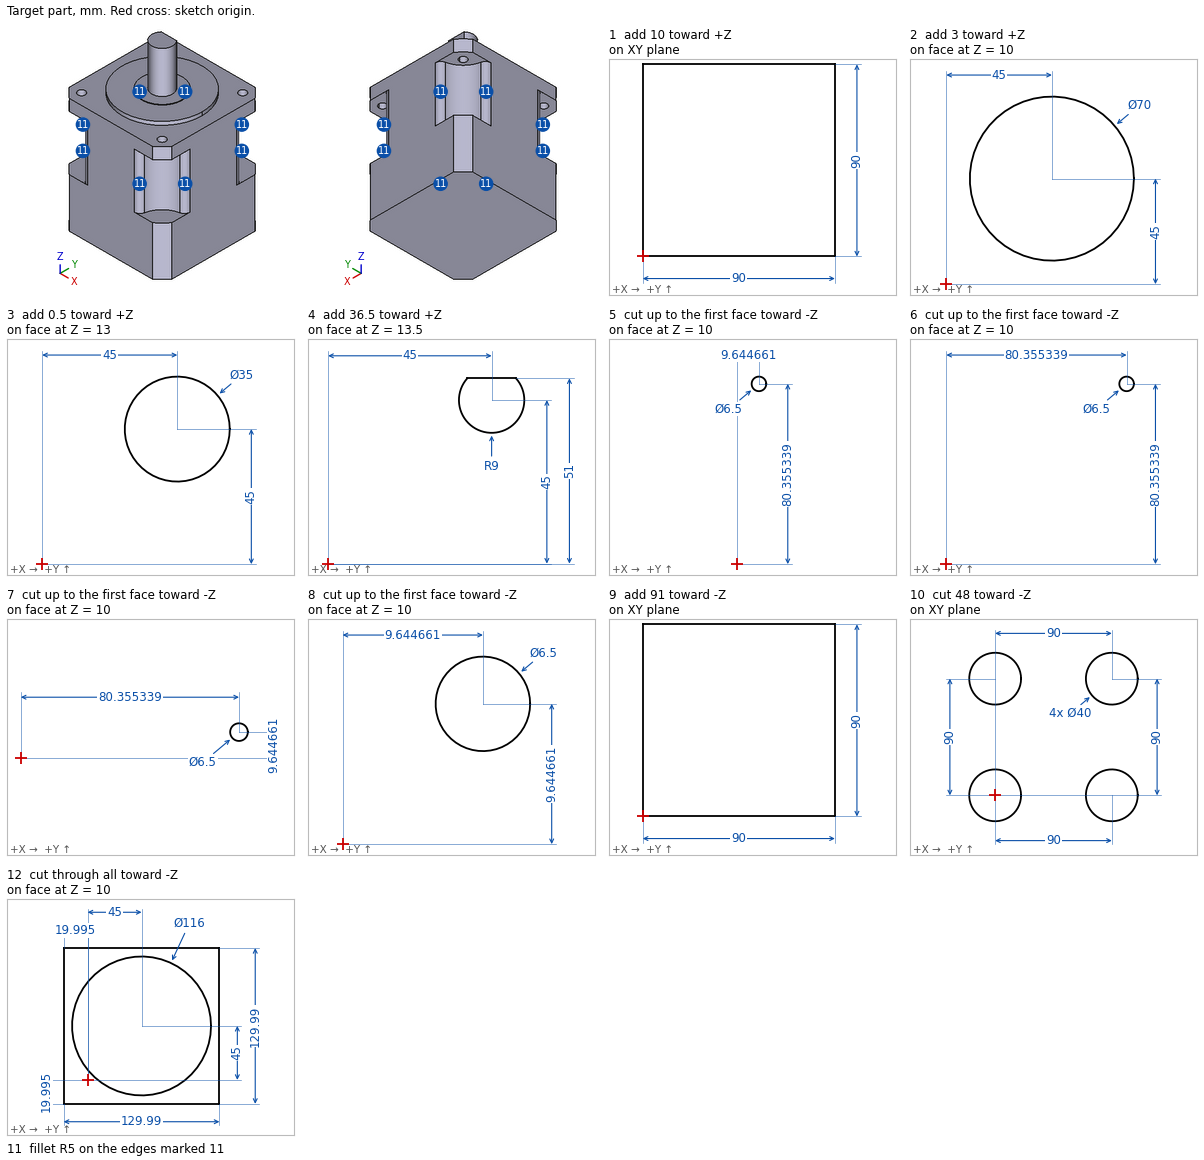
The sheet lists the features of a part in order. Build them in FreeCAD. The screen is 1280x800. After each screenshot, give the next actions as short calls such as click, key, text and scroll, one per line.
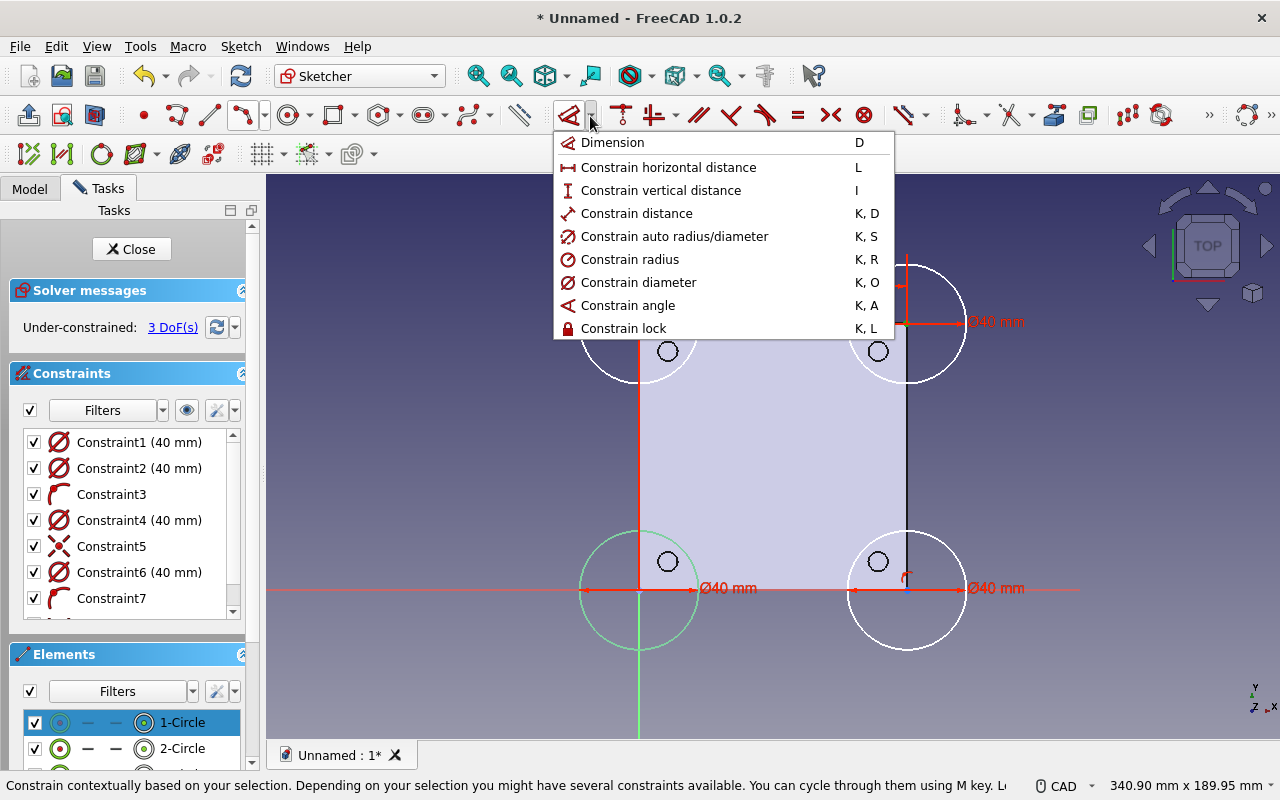
click(724, 190)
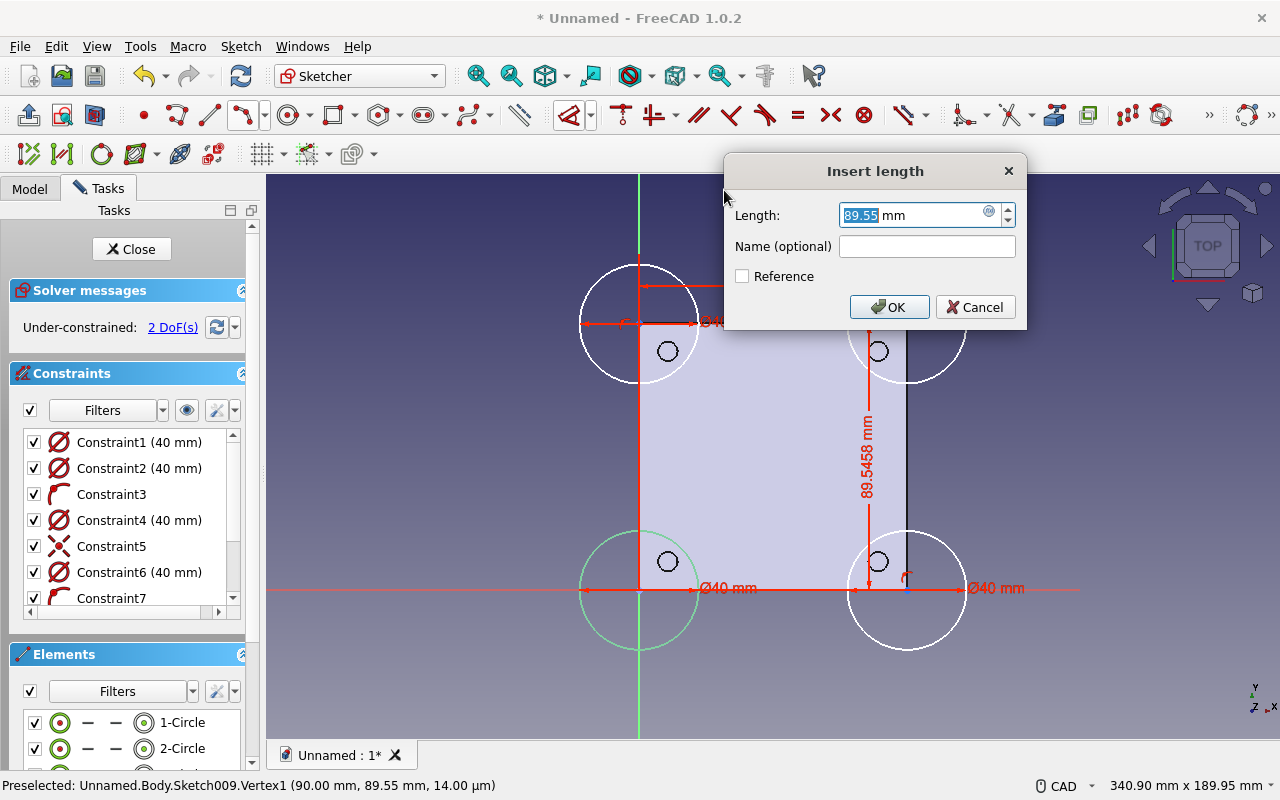
text(90)
key(Return)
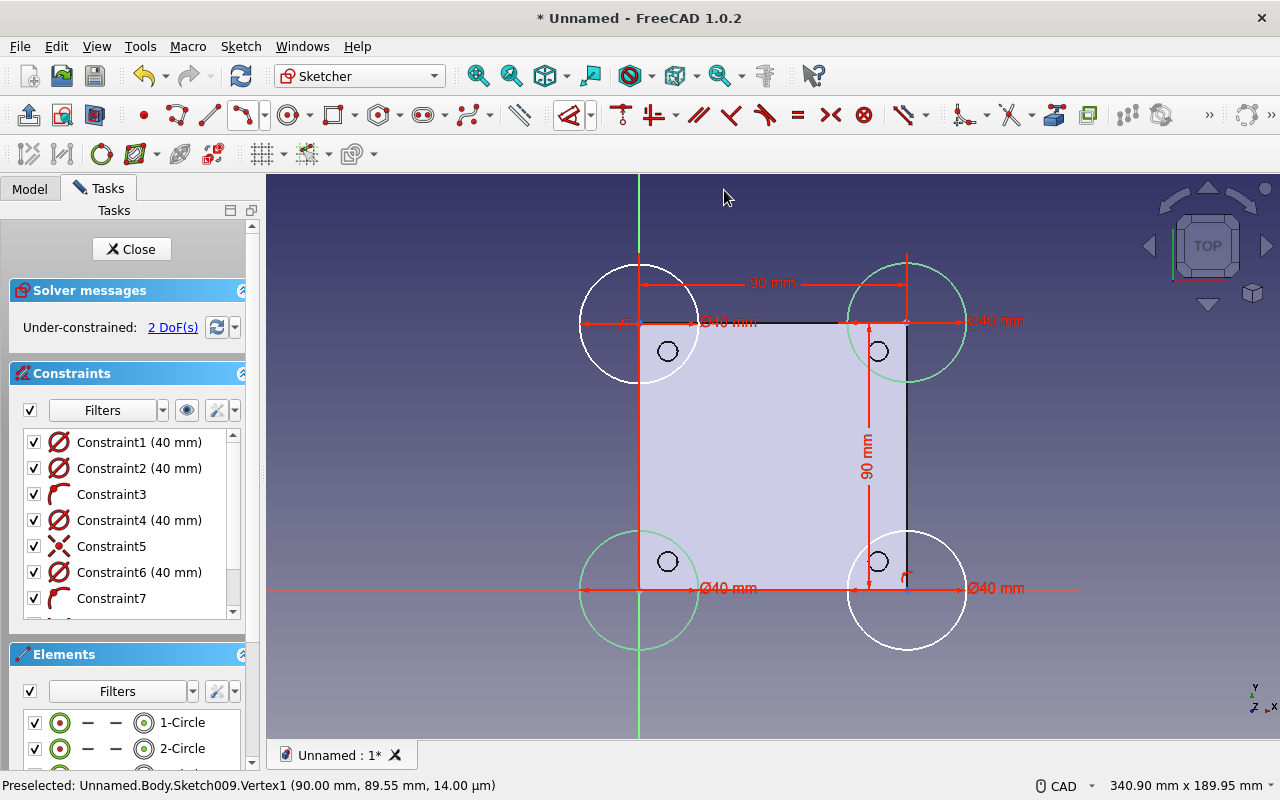
click(907, 590)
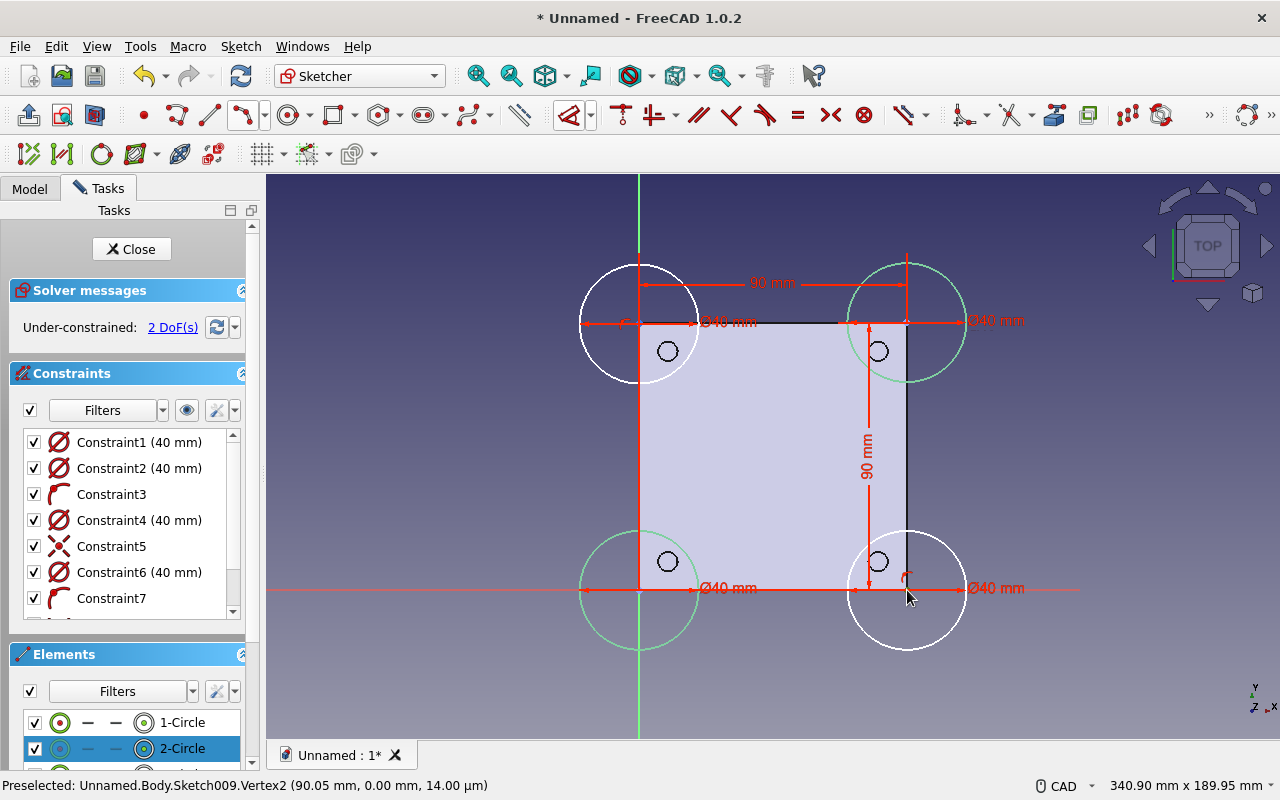
key(l)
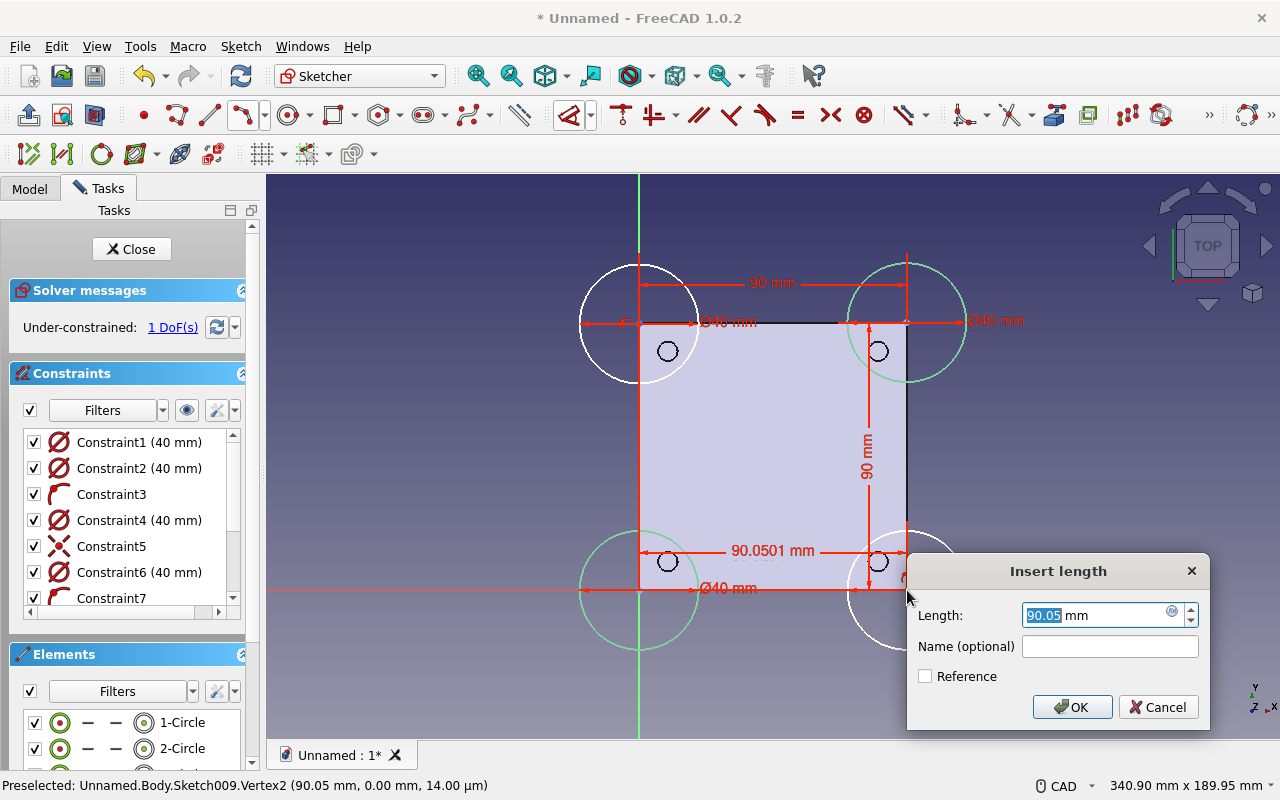
text(90)
key(Return)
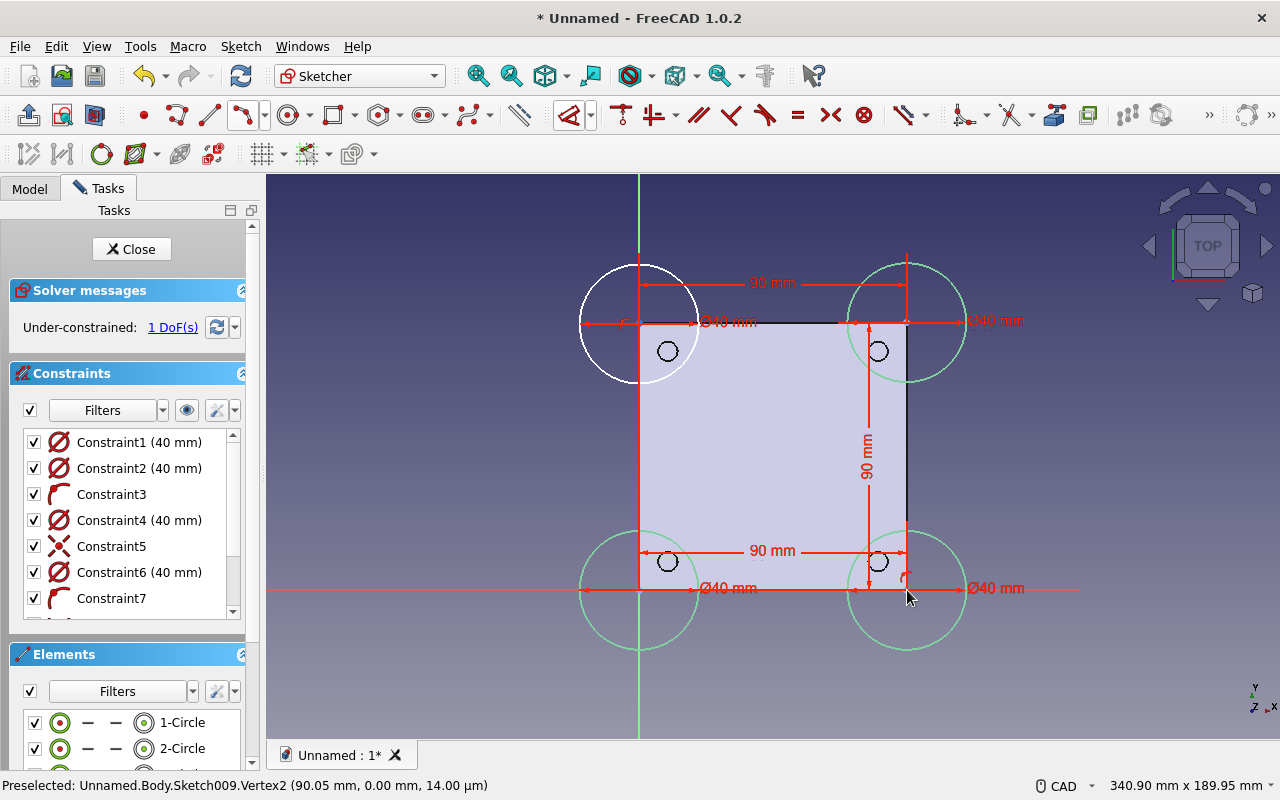
click(639, 324)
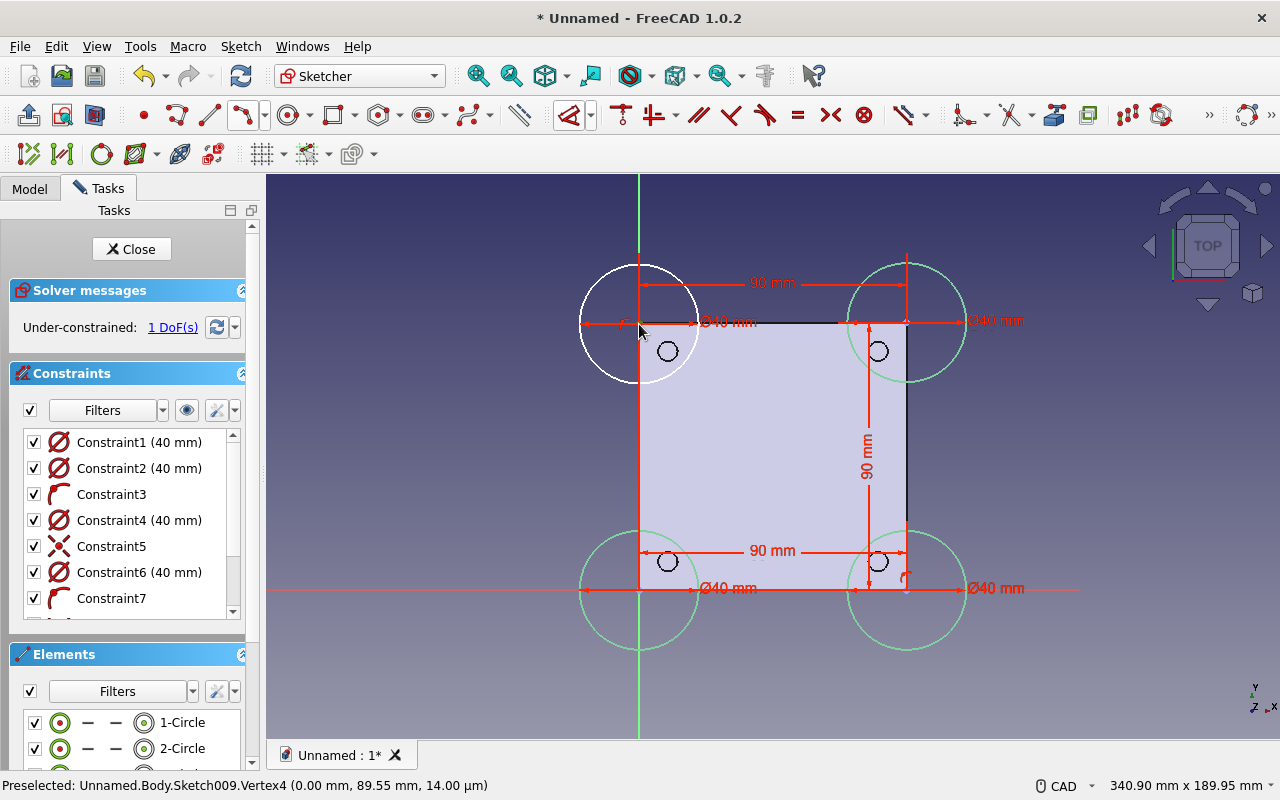
key(i)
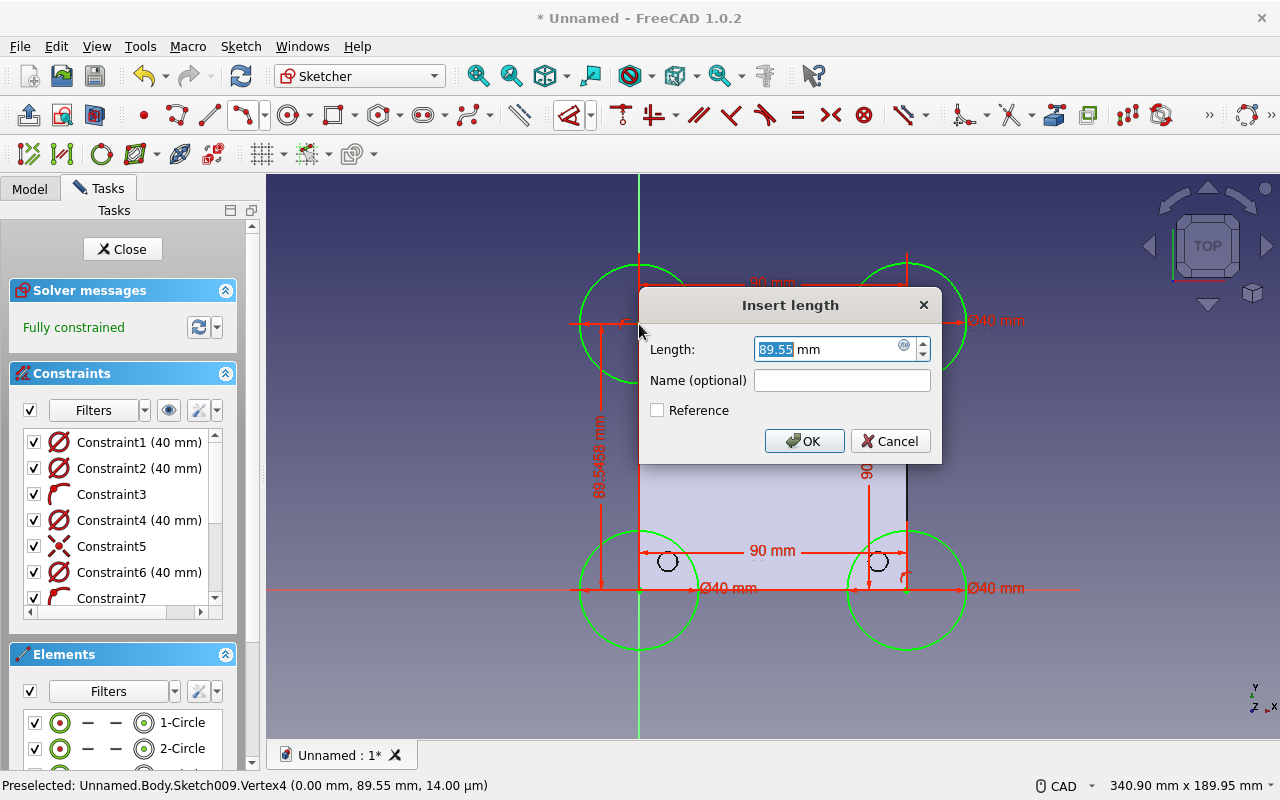
text(90)
key(Return)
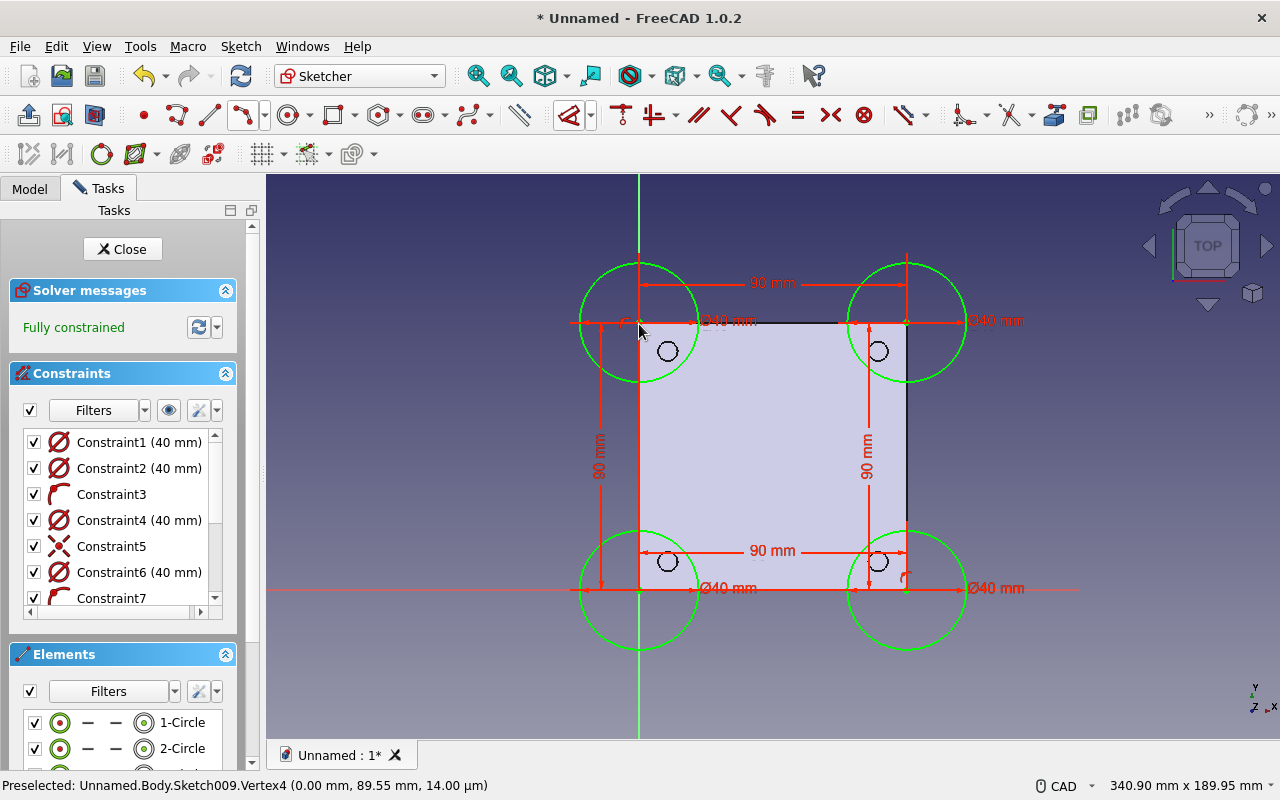
click(123, 249)